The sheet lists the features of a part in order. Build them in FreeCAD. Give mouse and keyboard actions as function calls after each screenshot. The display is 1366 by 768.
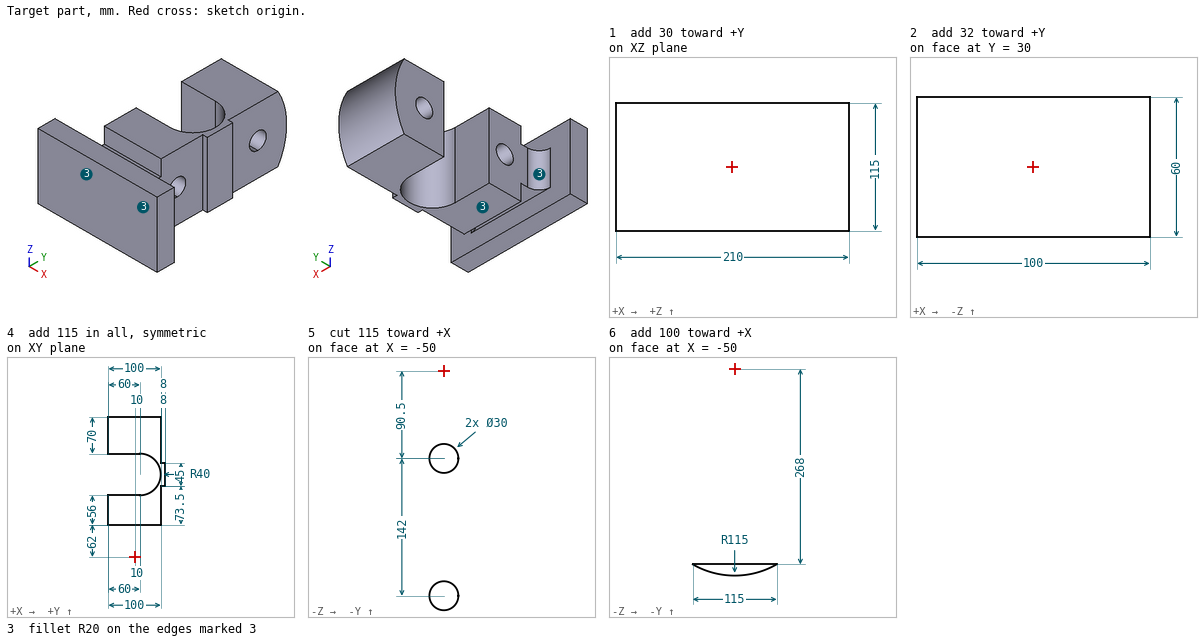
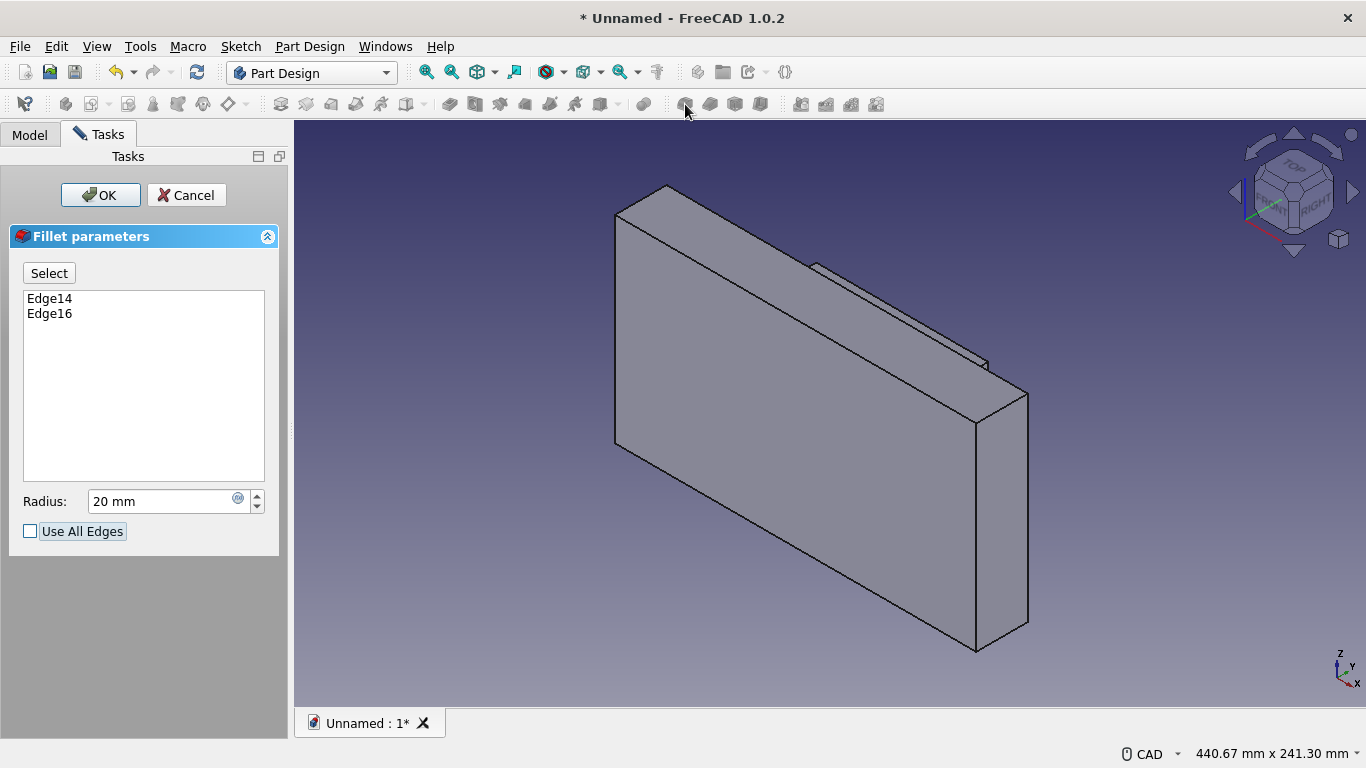
click(101, 195)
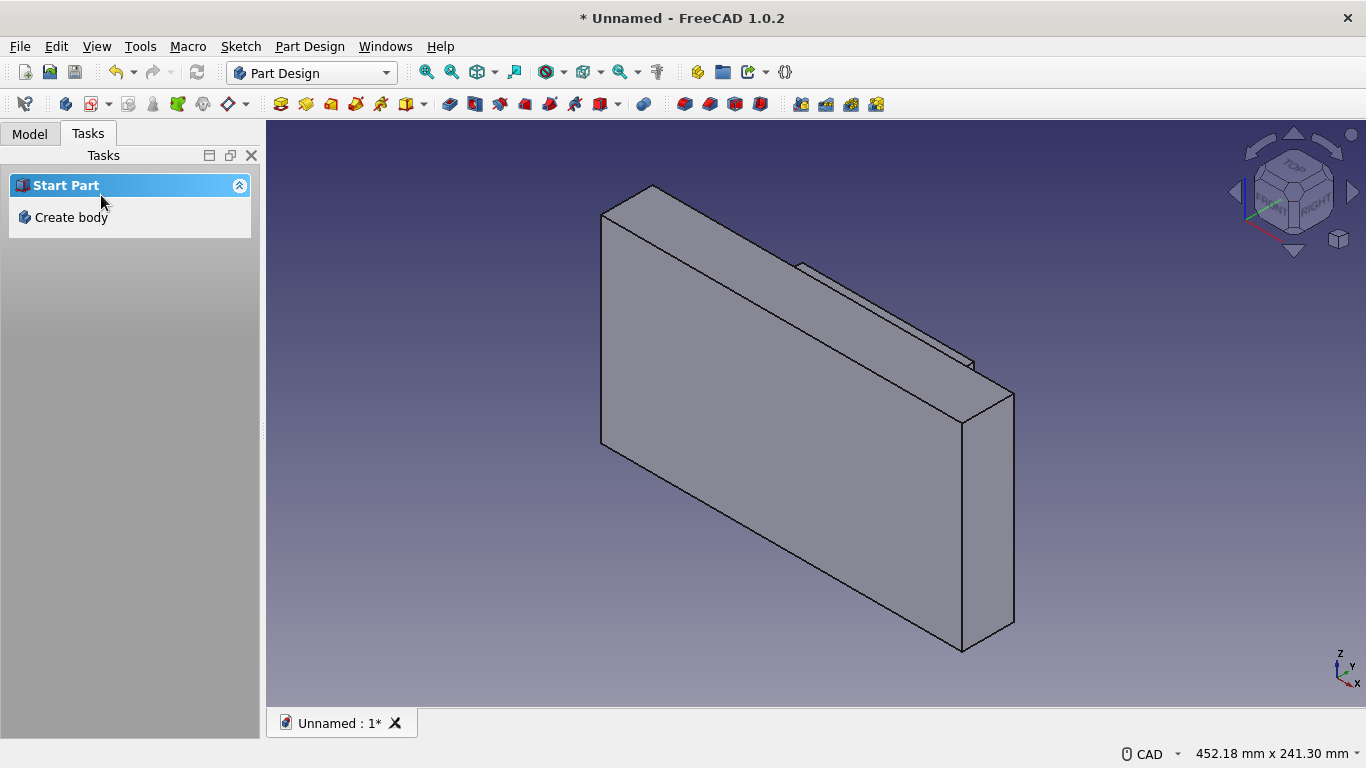
click(90, 104)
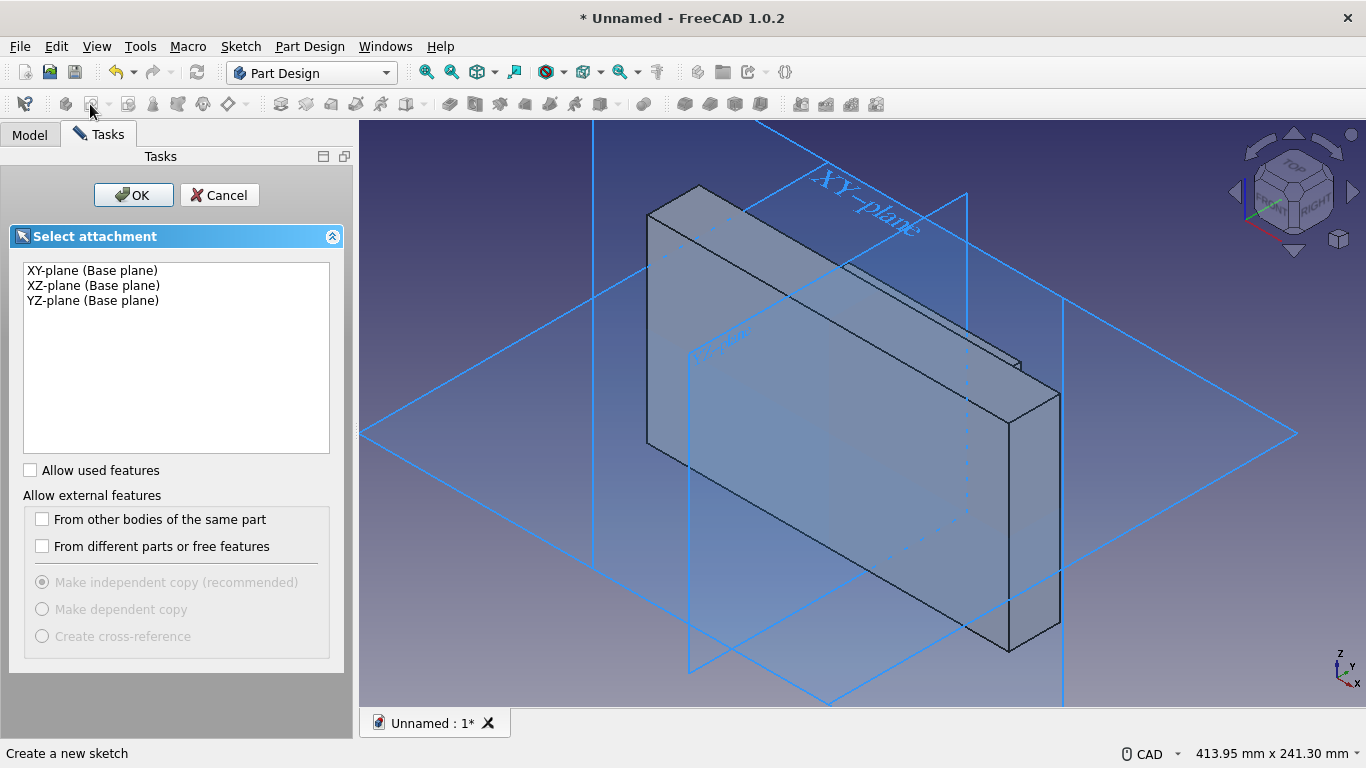
click(84, 270)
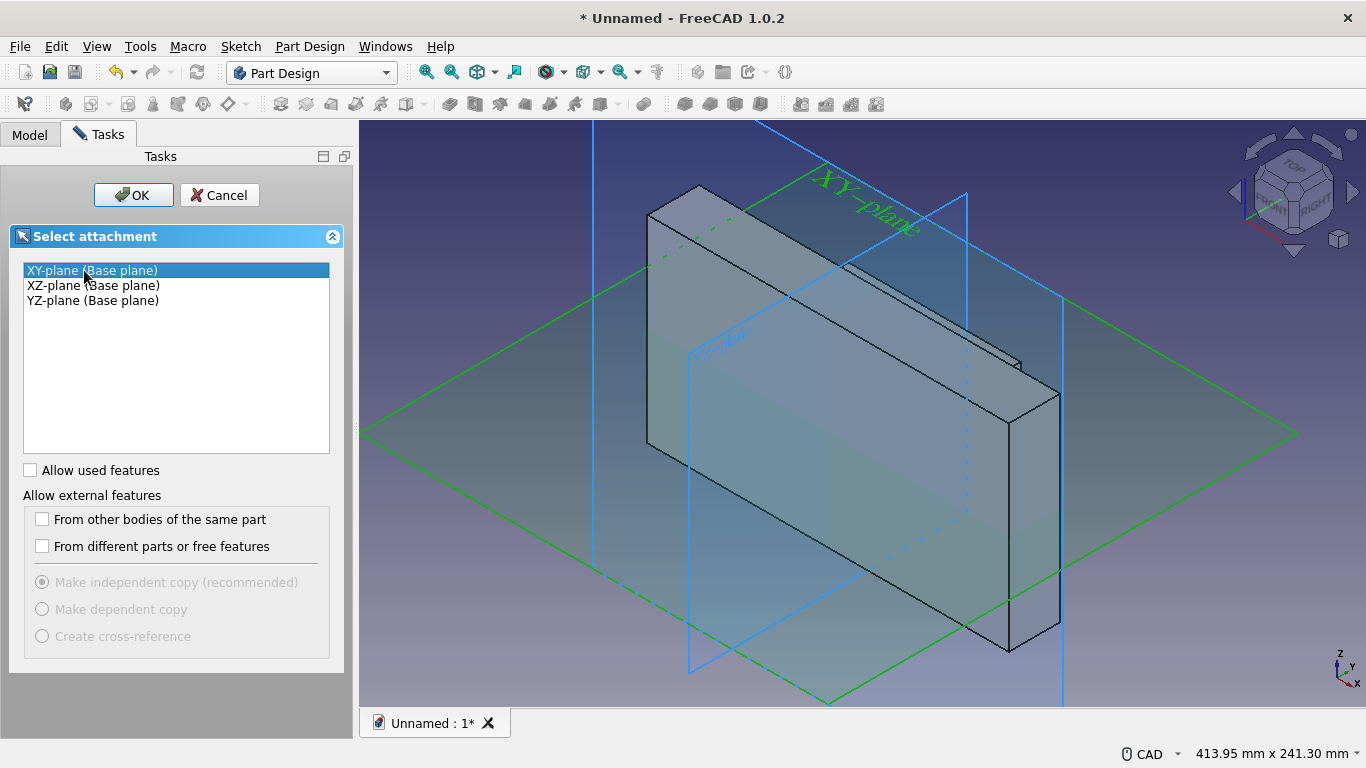
click(134, 195)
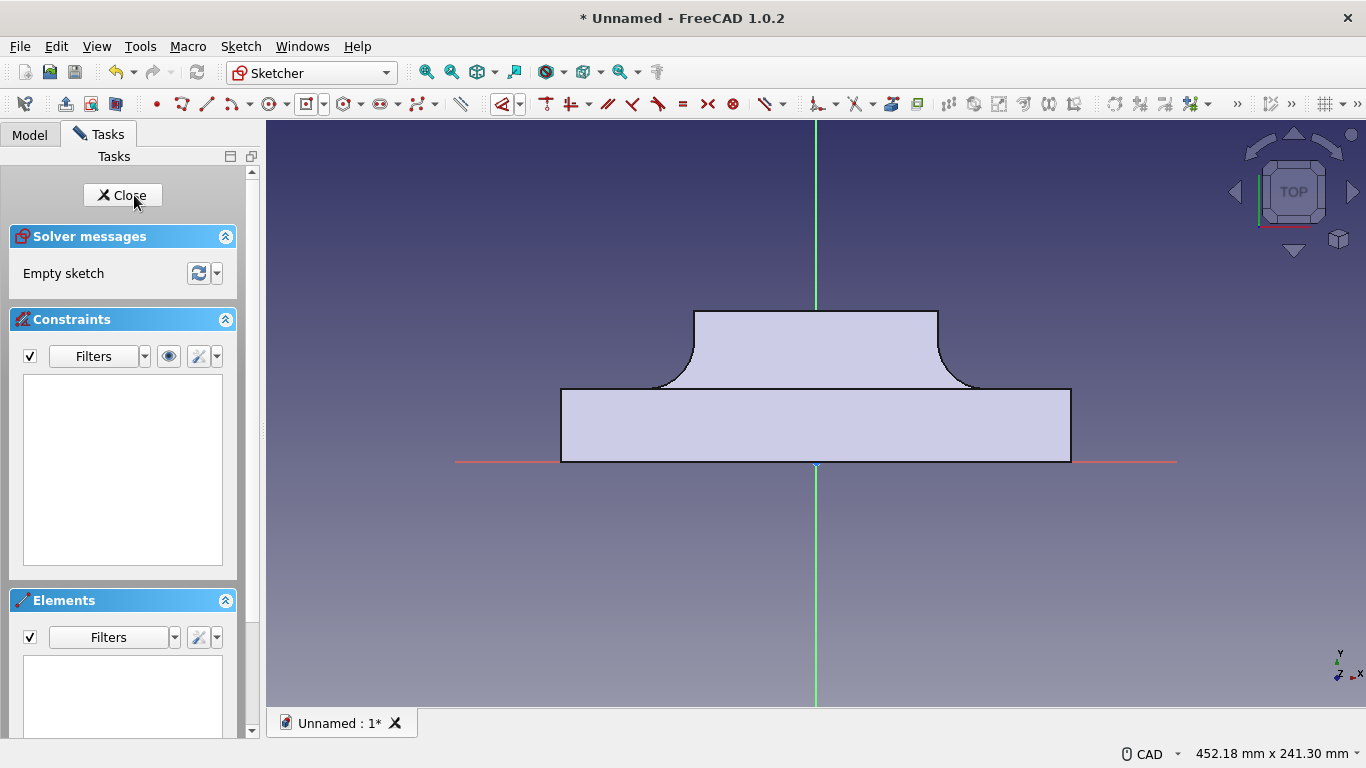
key(q)
key(s)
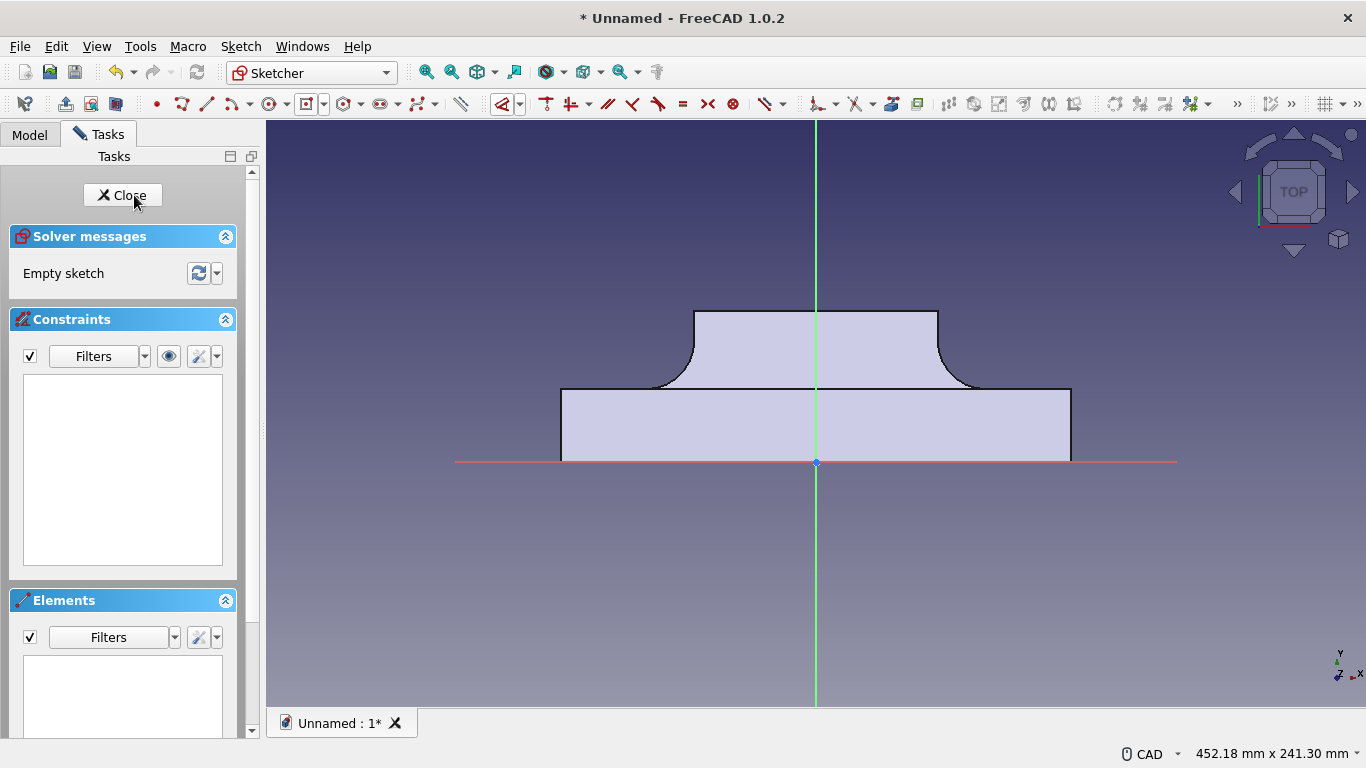
scroll(652, 679, down, 3)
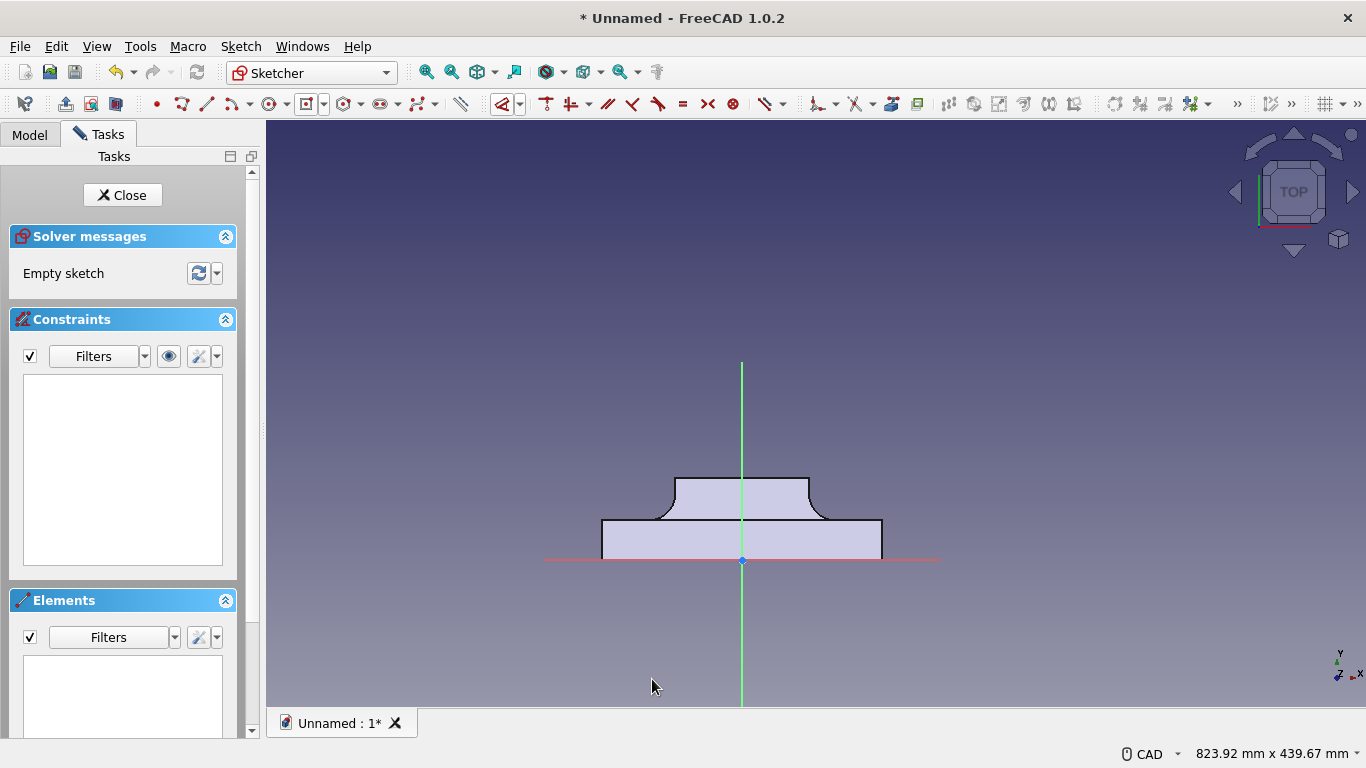
click(182, 104)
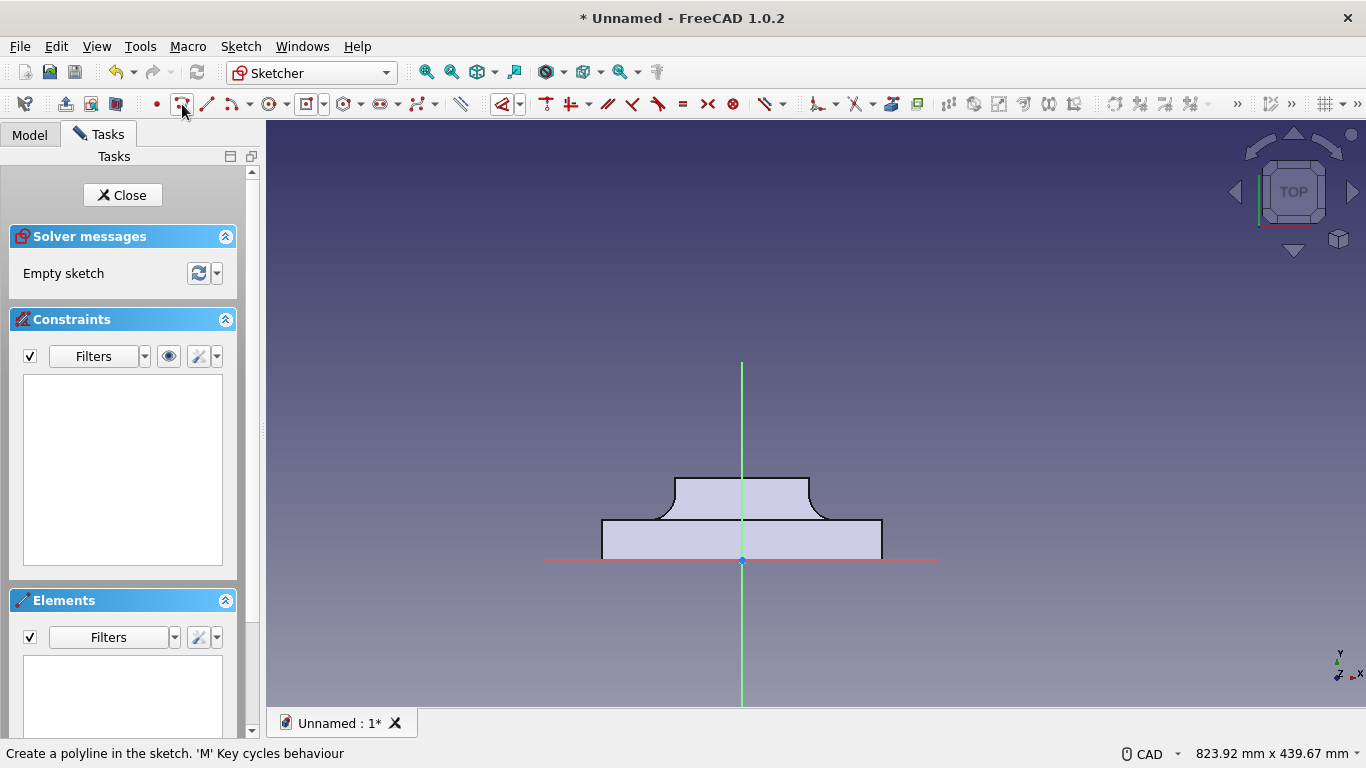
click(756, 403)
click(675, 403)
click(675, 478)
click(809, 478)
click(809, 380)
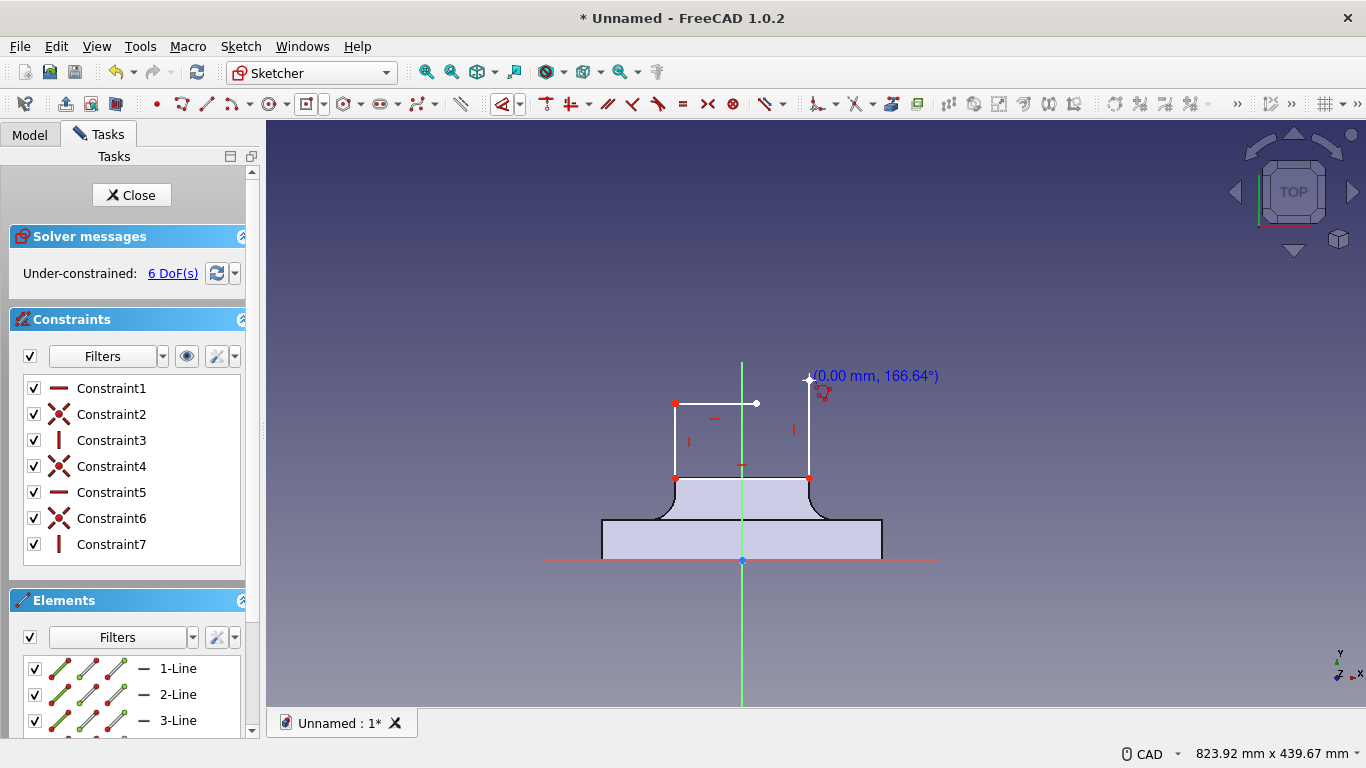
scroll(820, 380, up, 2)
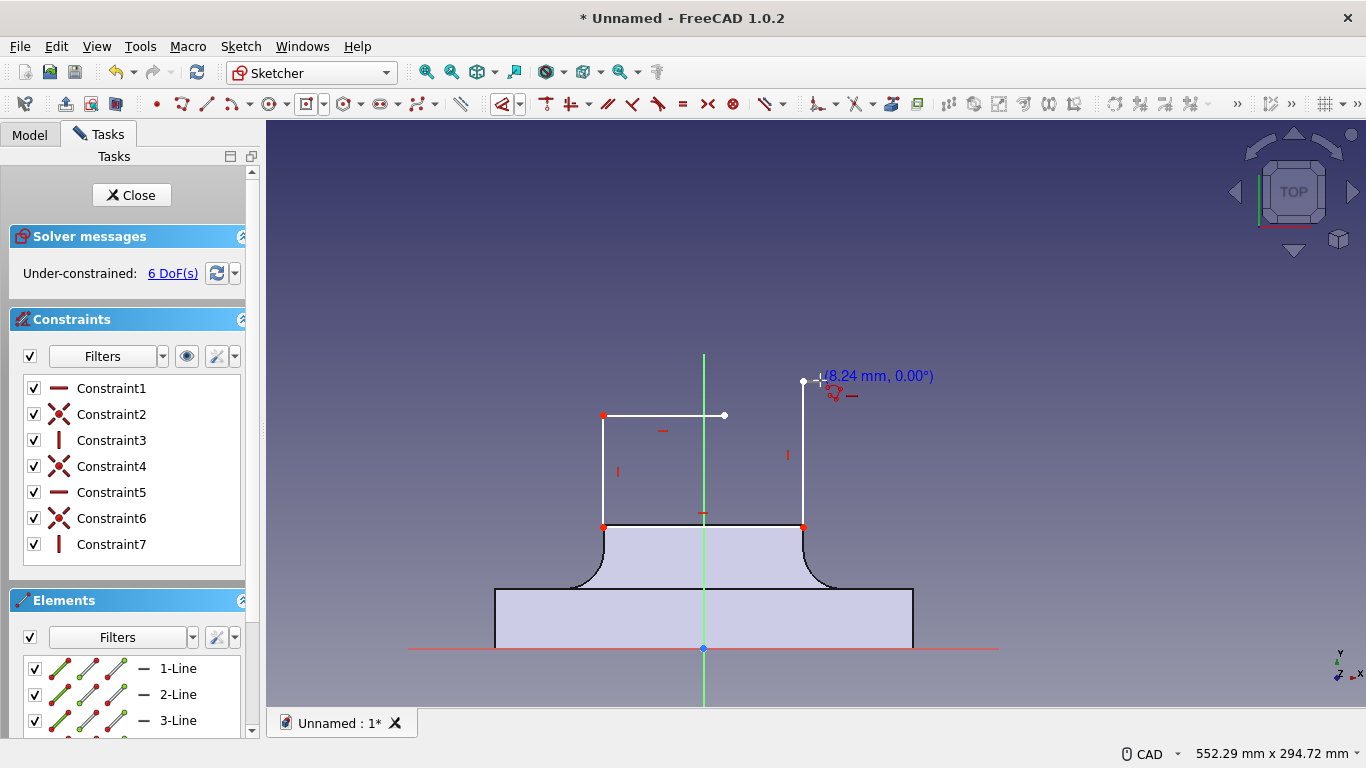
click(819, 380)
click(819, 289)
click(803, 289)